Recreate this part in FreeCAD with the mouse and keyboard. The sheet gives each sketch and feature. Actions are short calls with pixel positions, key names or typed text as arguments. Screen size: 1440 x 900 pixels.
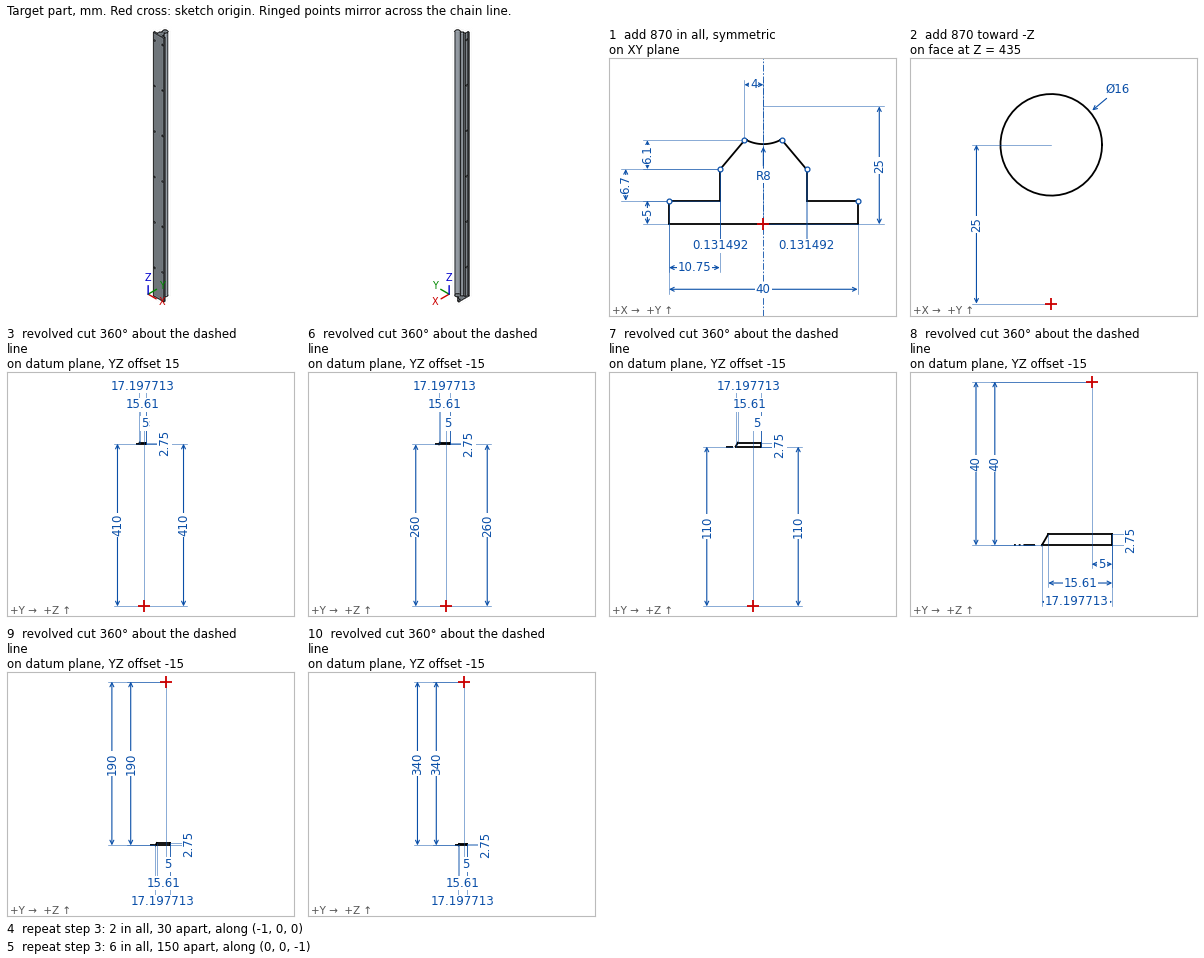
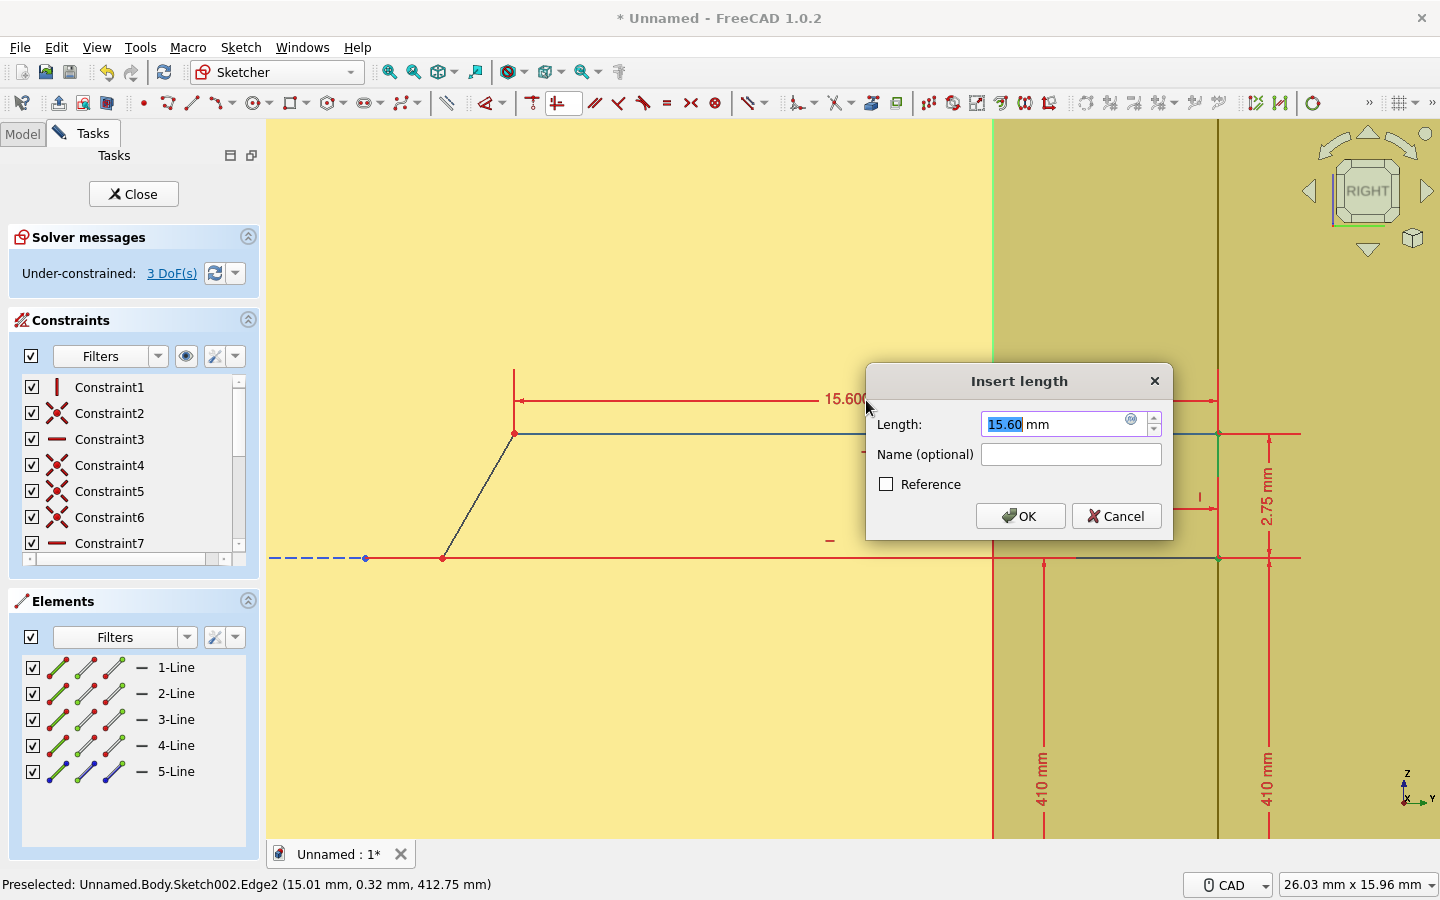
text(15.61)
key(Return)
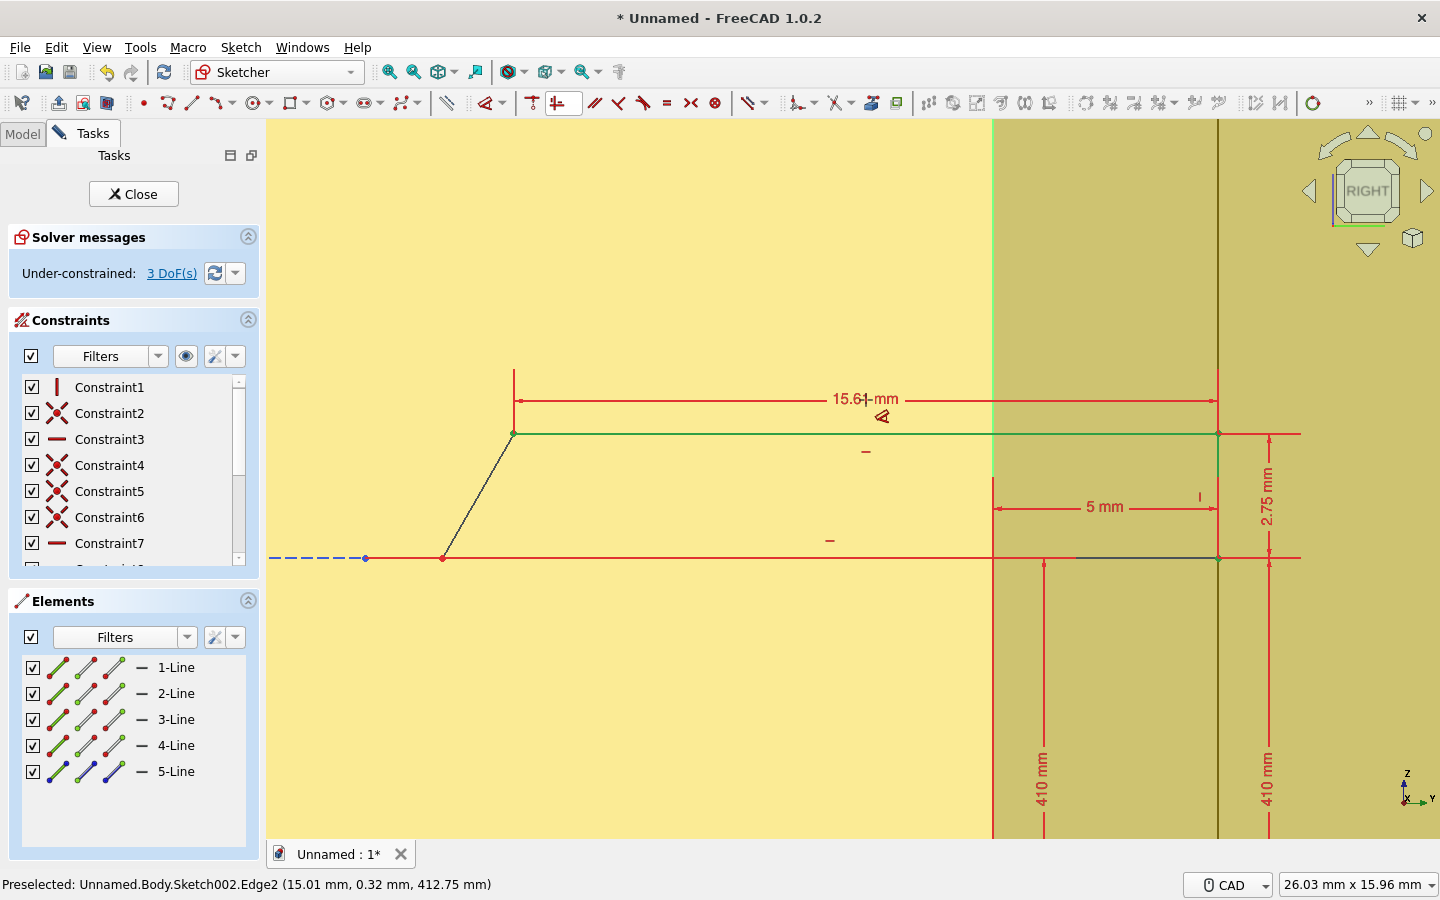
click(675, 558)
click(830, 592)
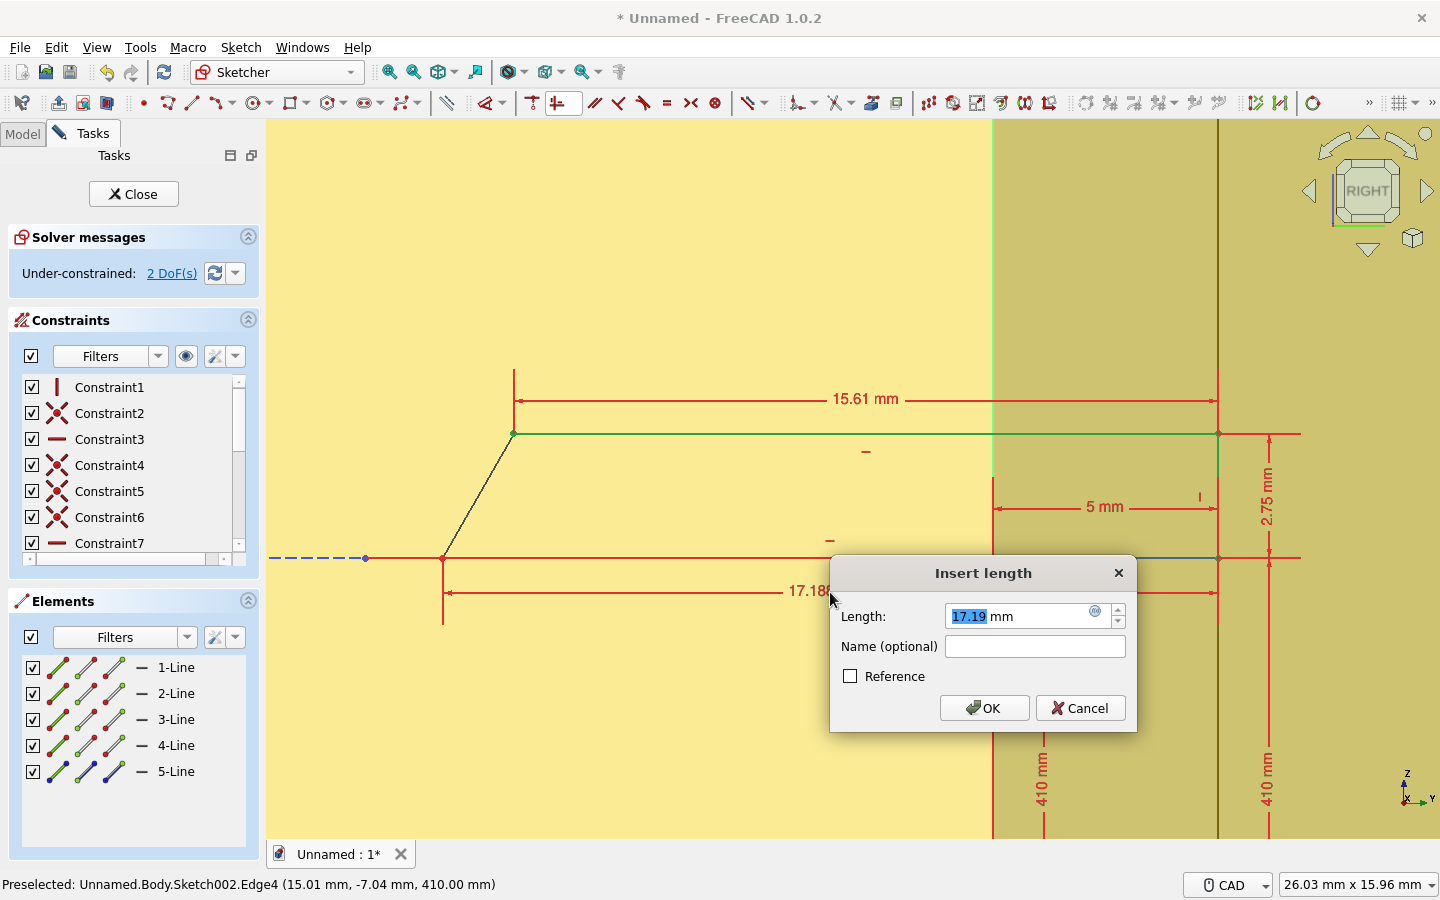
text(17.197713)
key(Return)
key(Escape)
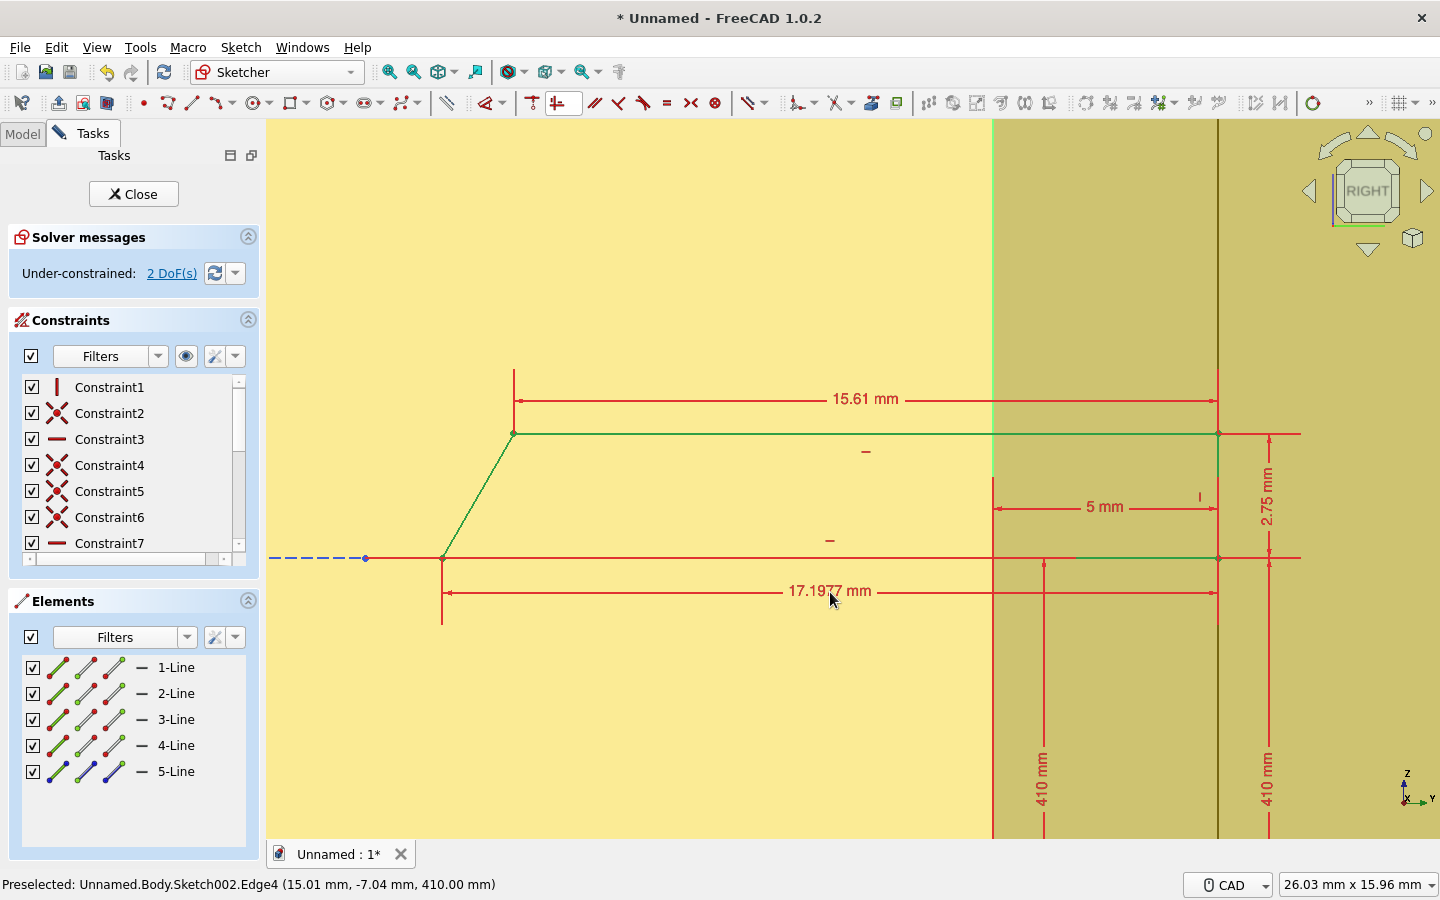
click(134, 194)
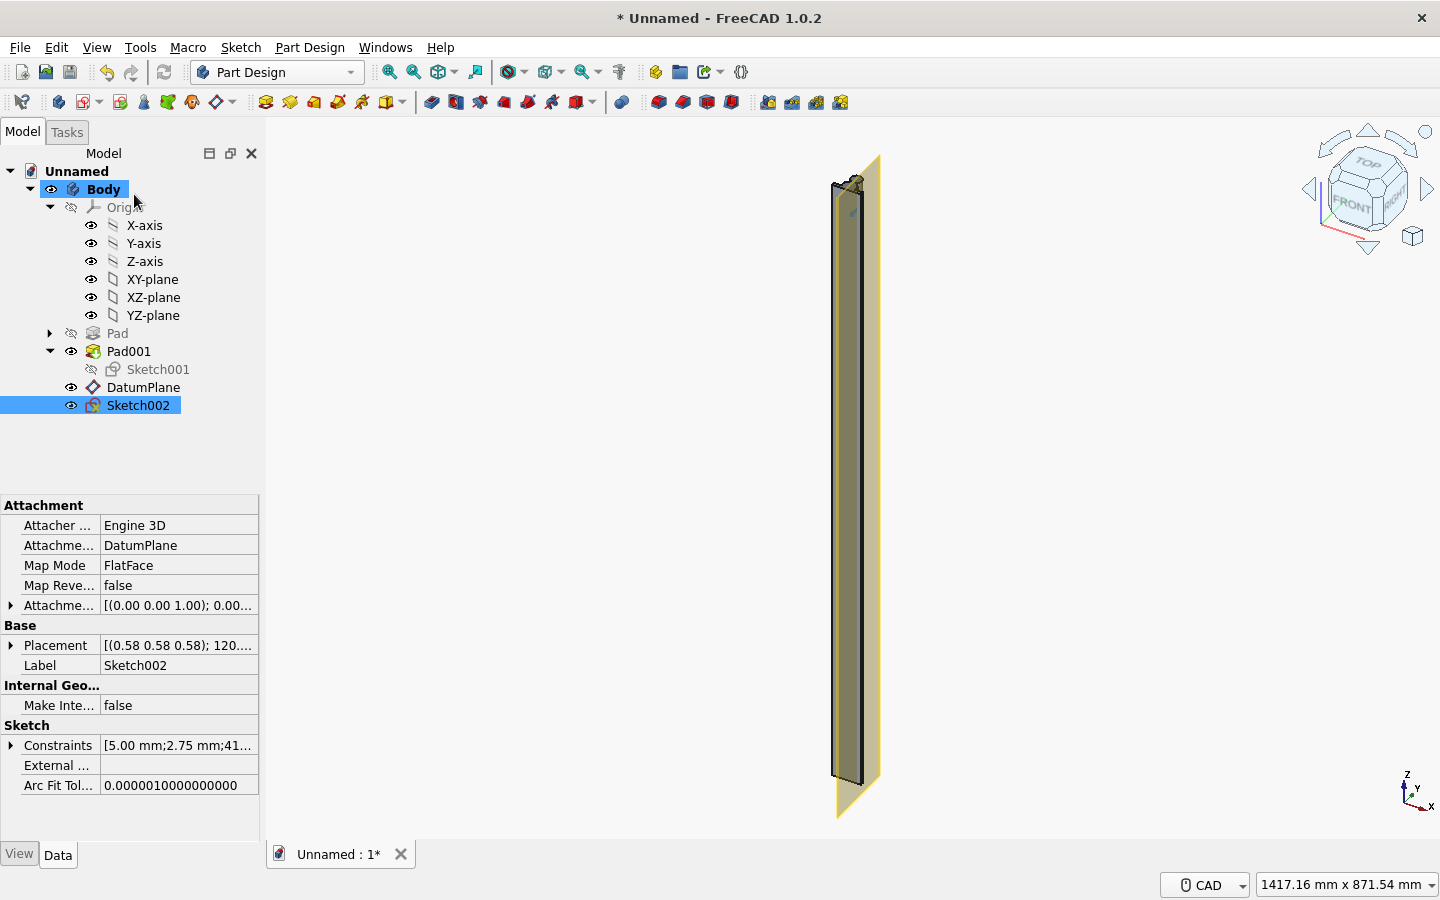
click(480, 102)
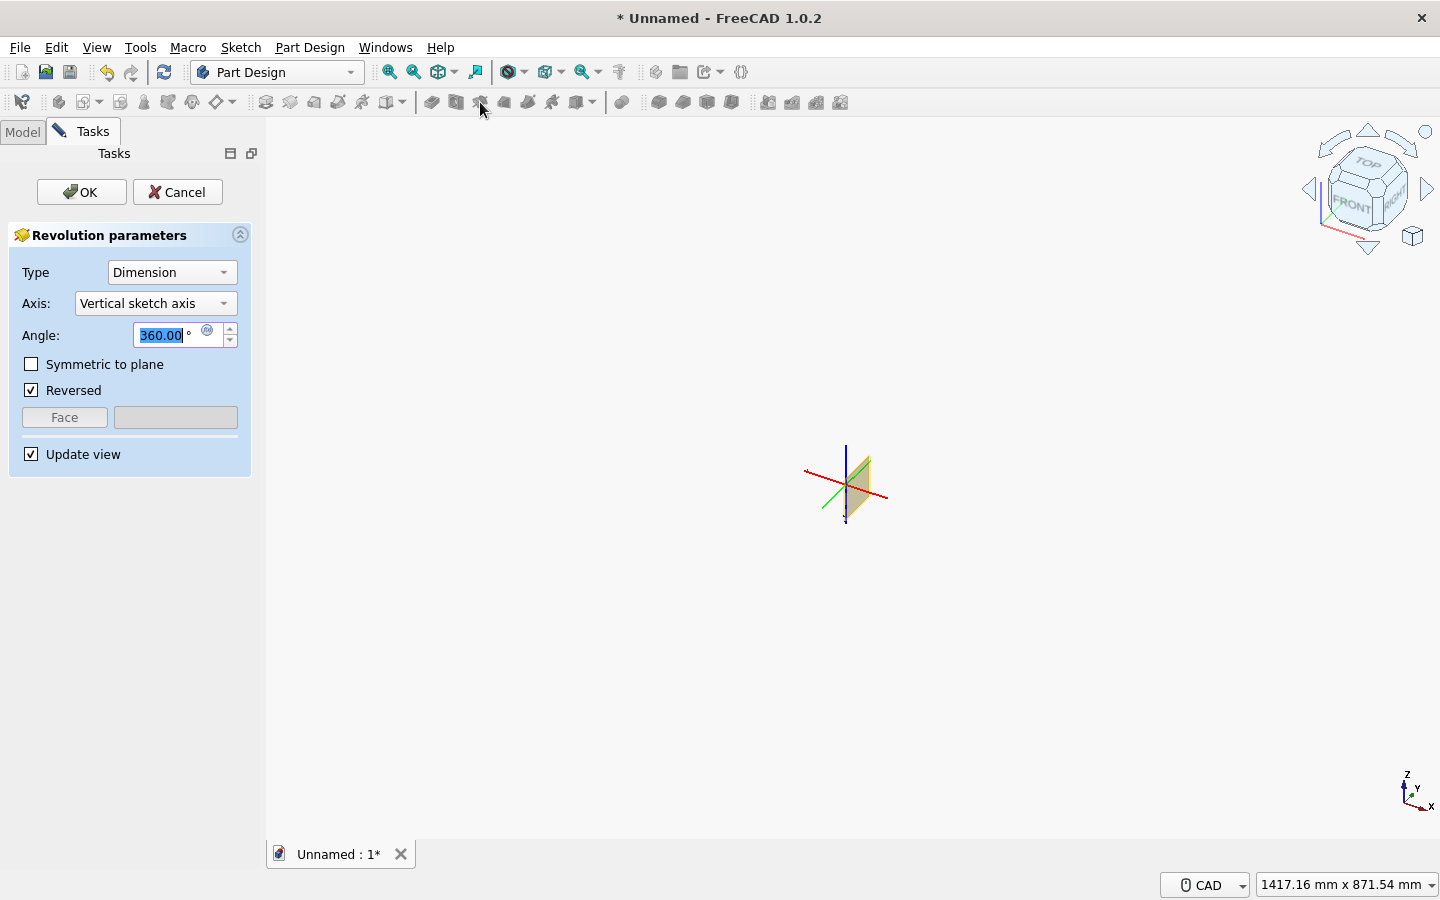
click(156, 304)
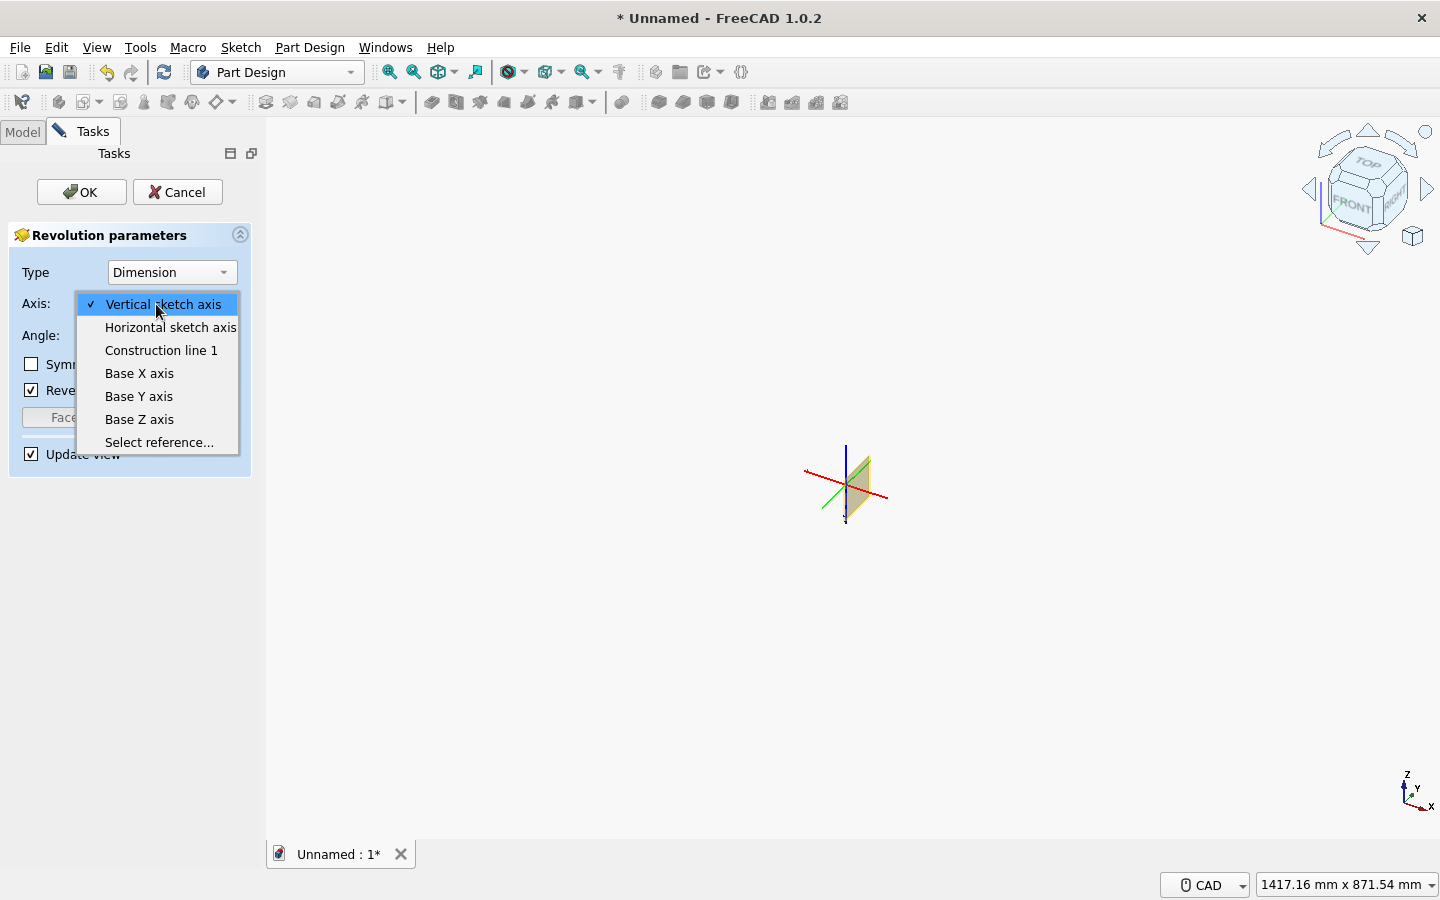
click(156, 350)